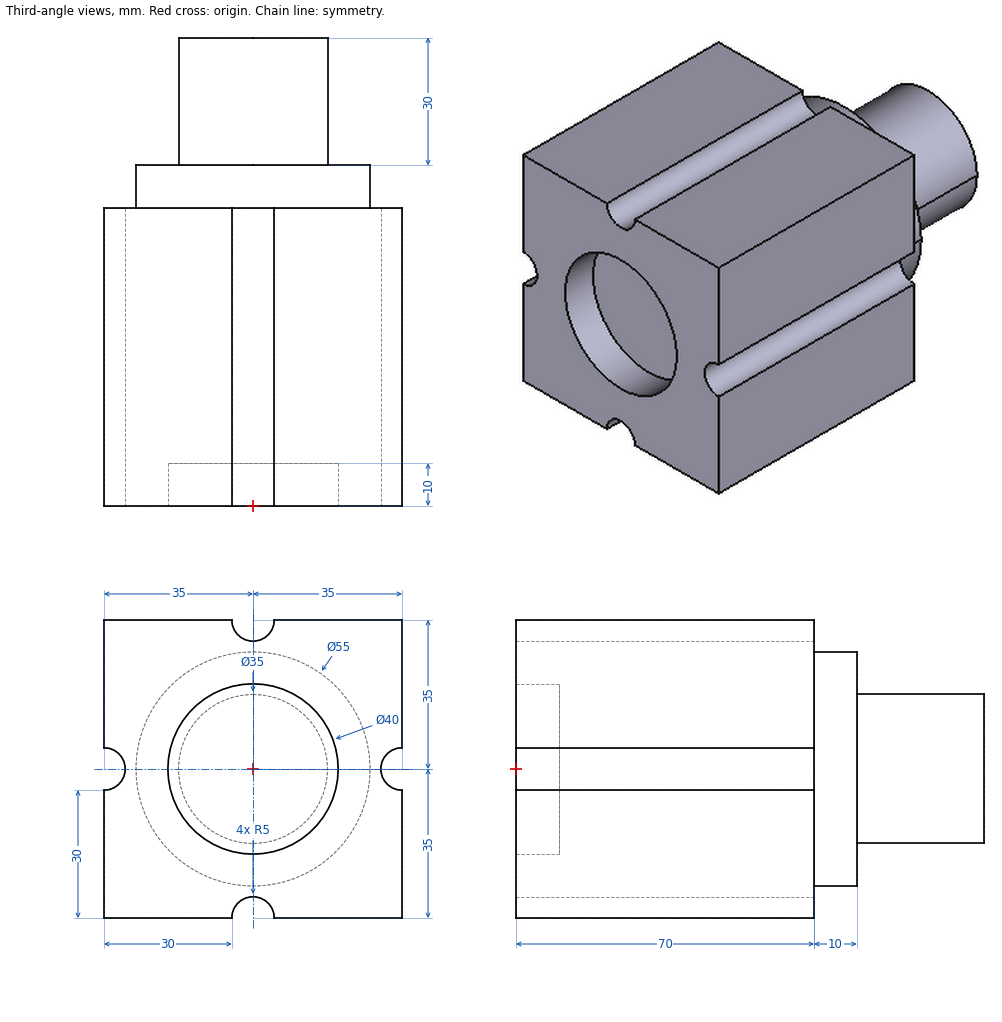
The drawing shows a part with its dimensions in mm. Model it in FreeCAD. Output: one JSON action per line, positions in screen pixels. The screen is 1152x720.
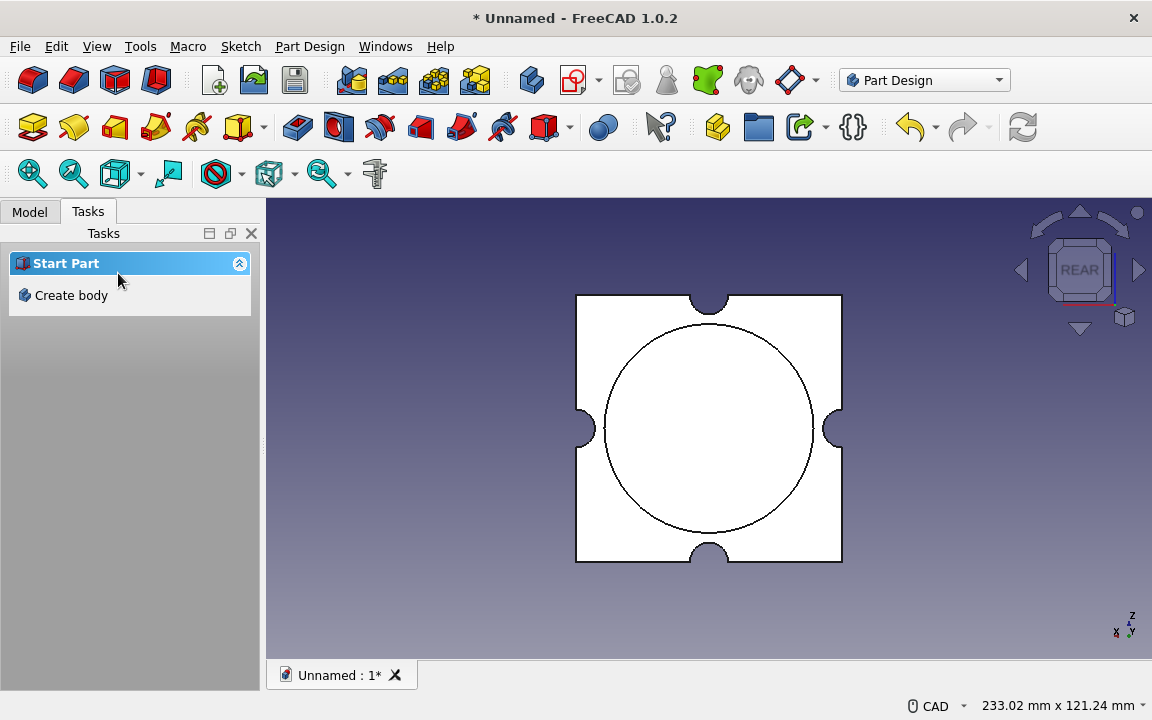
{"action": "left_click", "coordinate": [709, 428]}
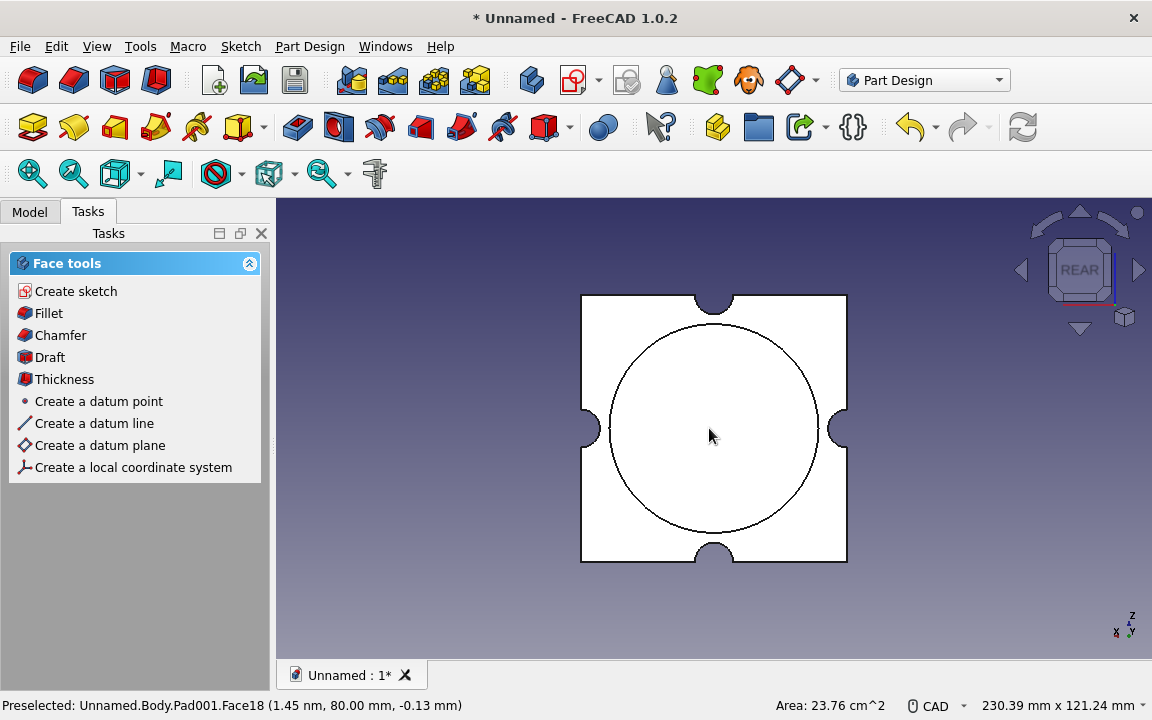
{"action": "left_click", "coordinate": [572, 80]}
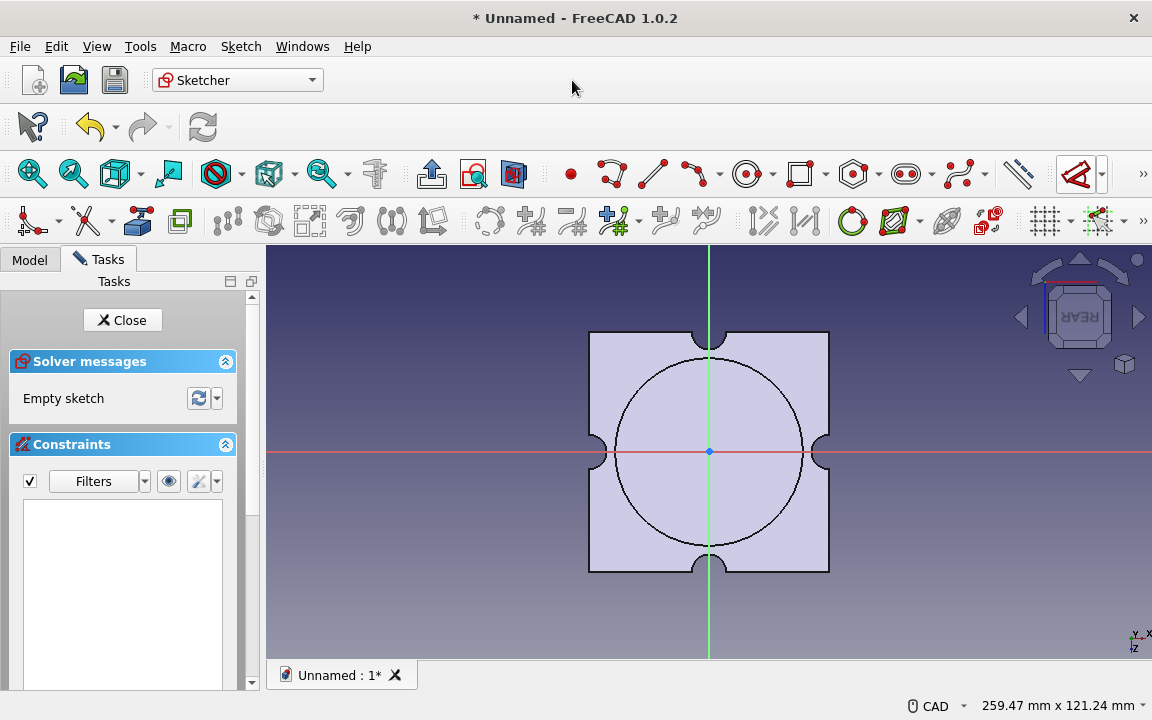
{"action": "scroll", "coordinate": [765, 452], "scroll_direction": "up", "scroll_amount": 4}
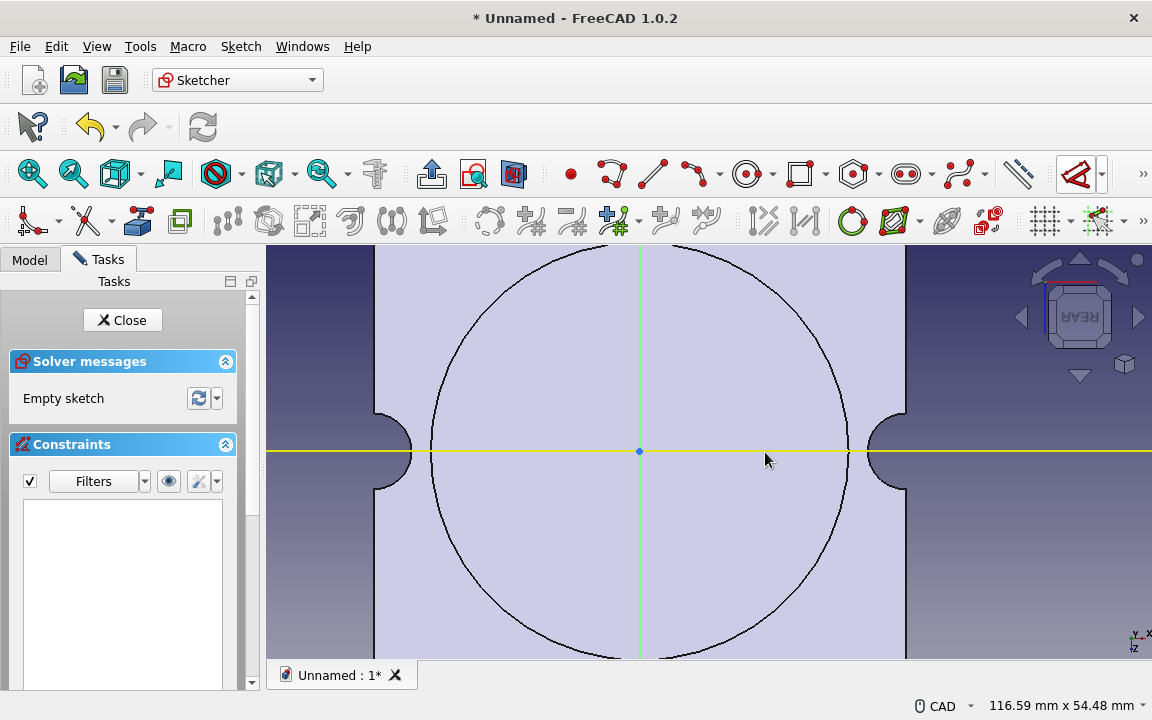
{"action": "left_click", "coordinate": [746, 174]}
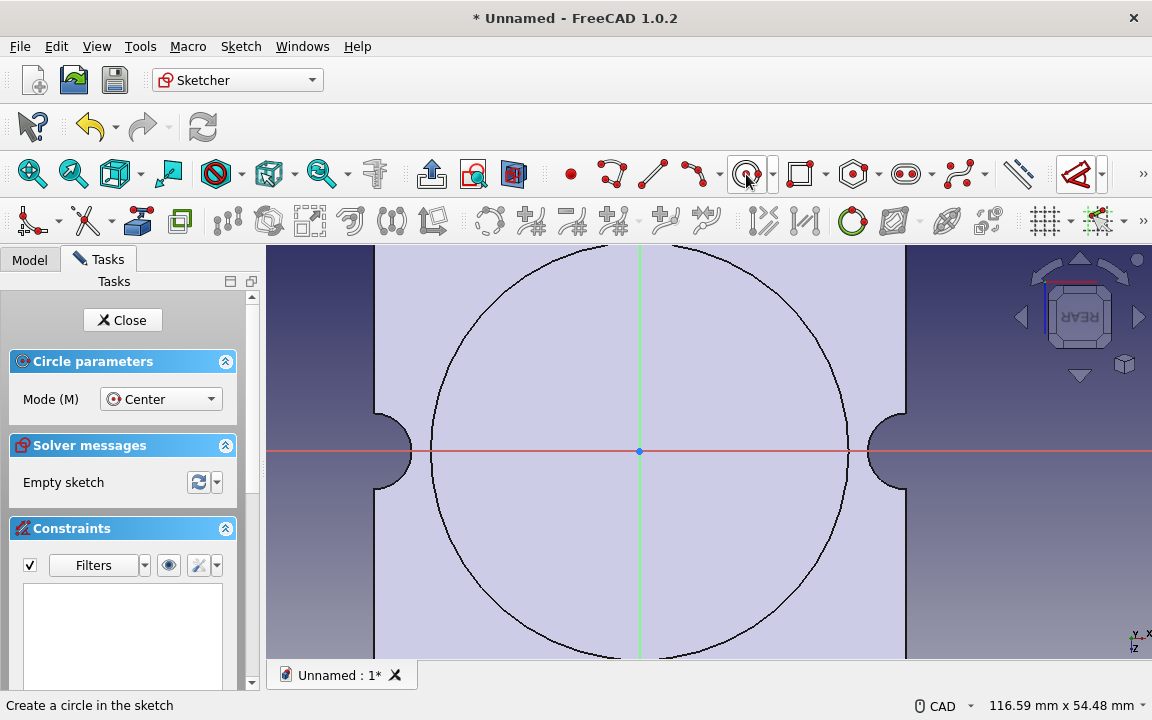
{"action": "left_click", "coordinate": [640, 451]}
{"action": "mouse_move", "coordinate": [734, 357]}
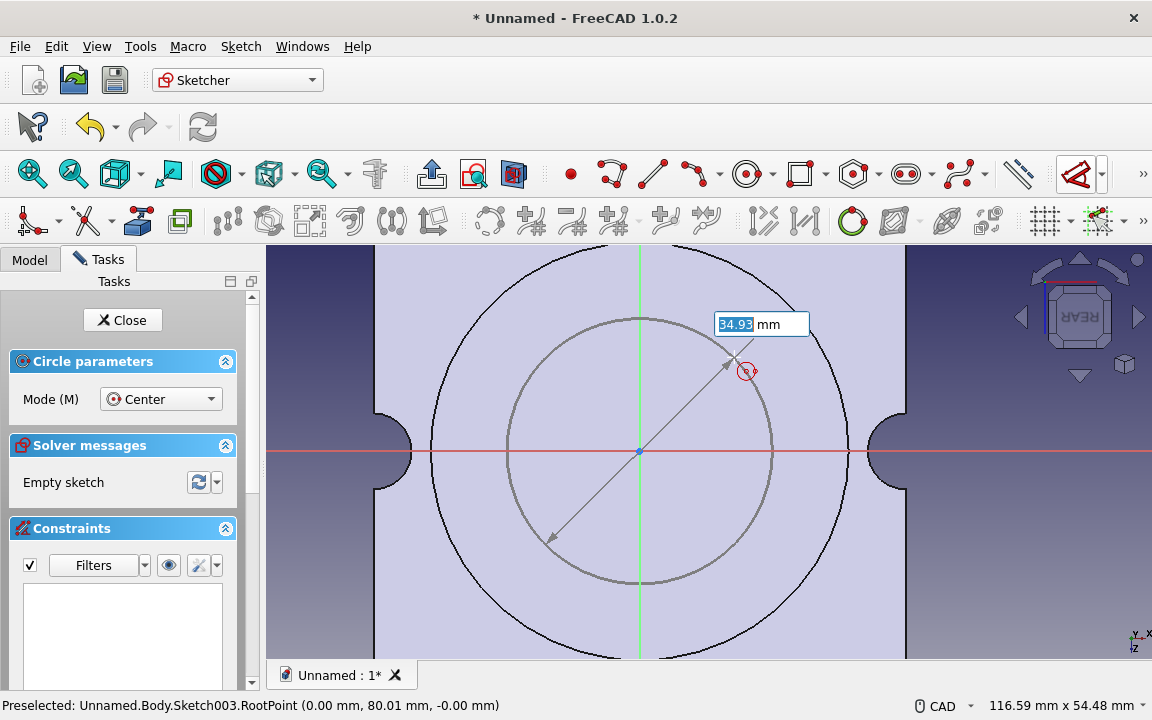
{"action": "type", "text": "35"}
{"action": "key", "text": "Return"}
{"action": "key", "text": "Escape"}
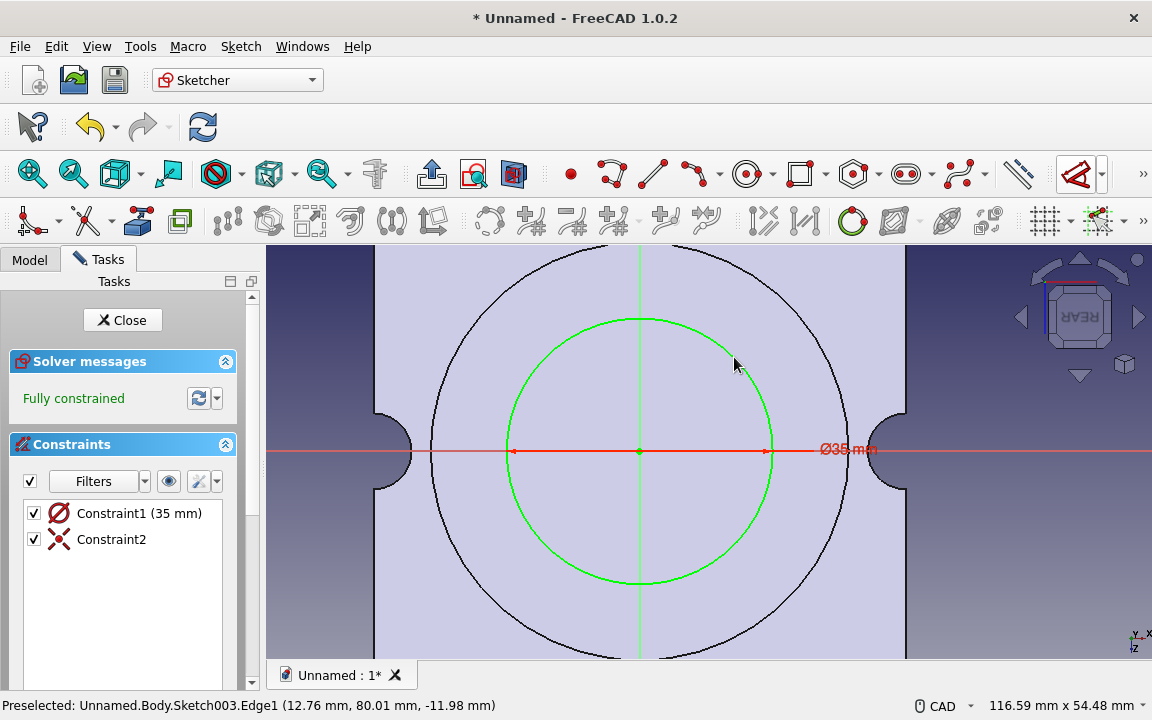
{"action": "left_click", "coordinate": [123, 320]}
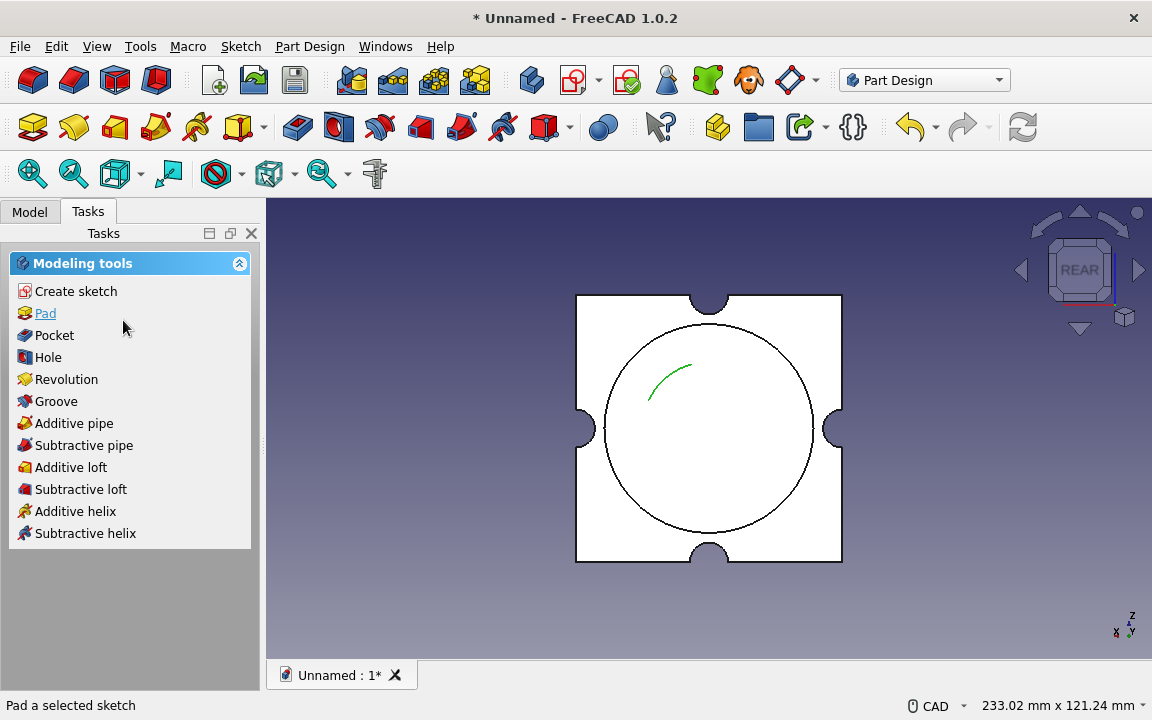
{"action": "left_click", "coordinate": [33, 128]}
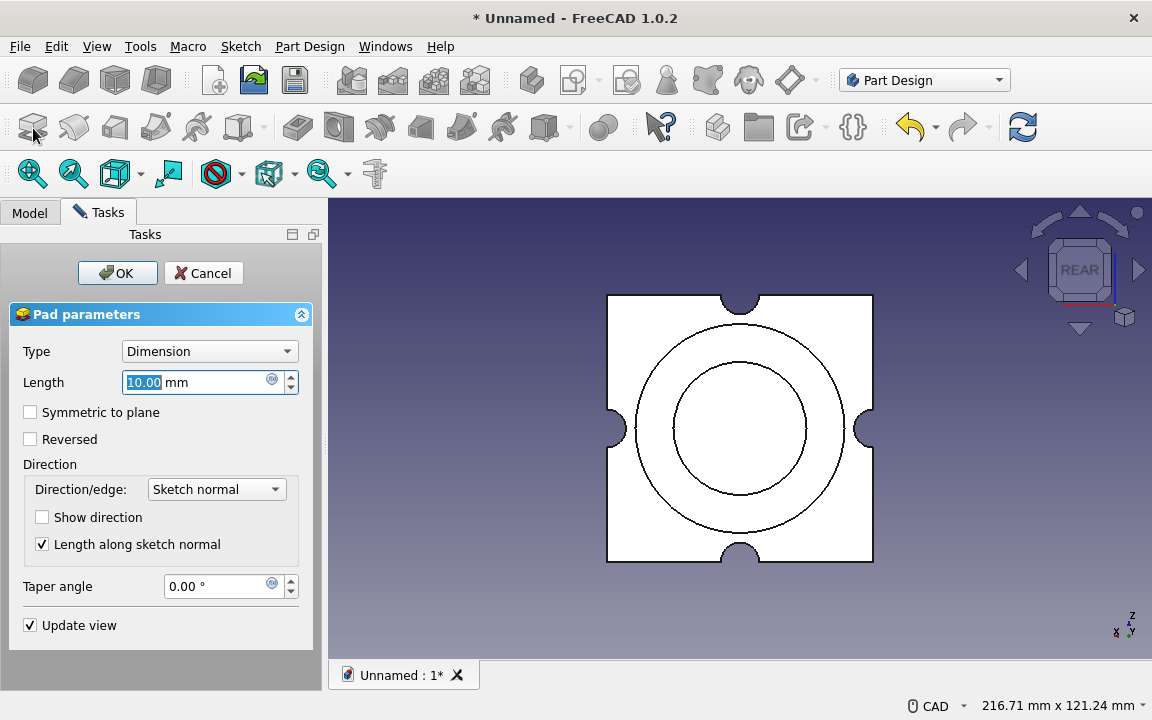
{"action": "type", "text": "30"}
{"action": "key", "text": "Tab"}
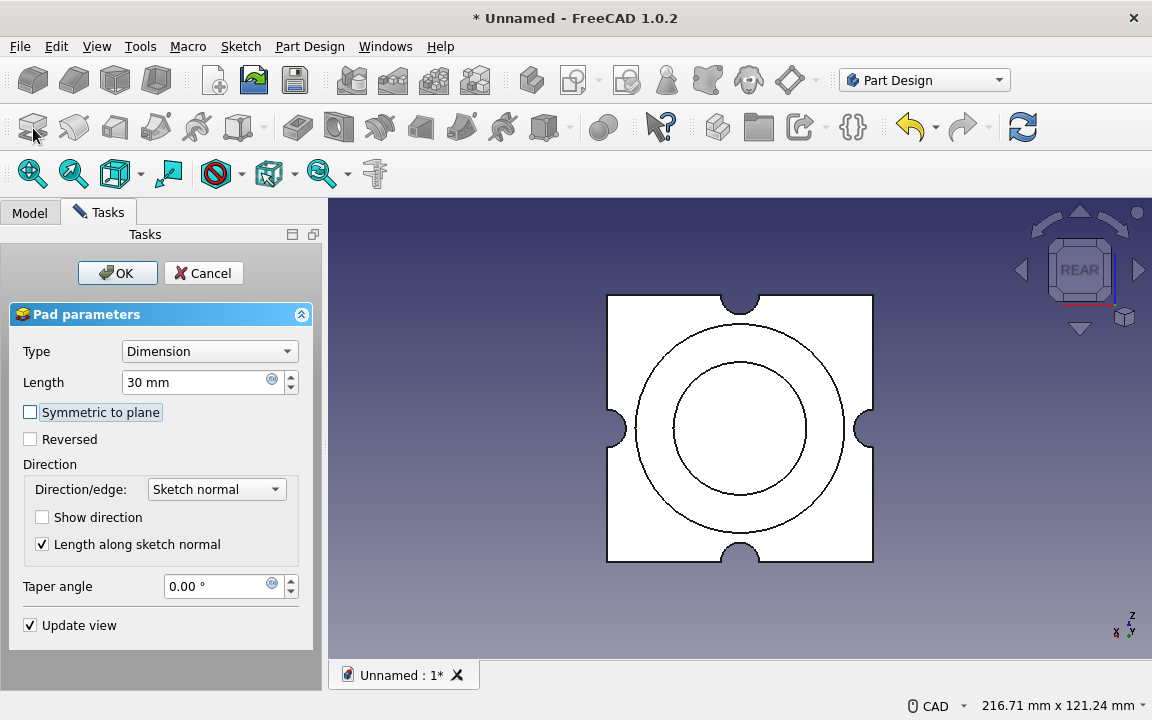
{"action": "left_click", "coordinate": [118, 273]}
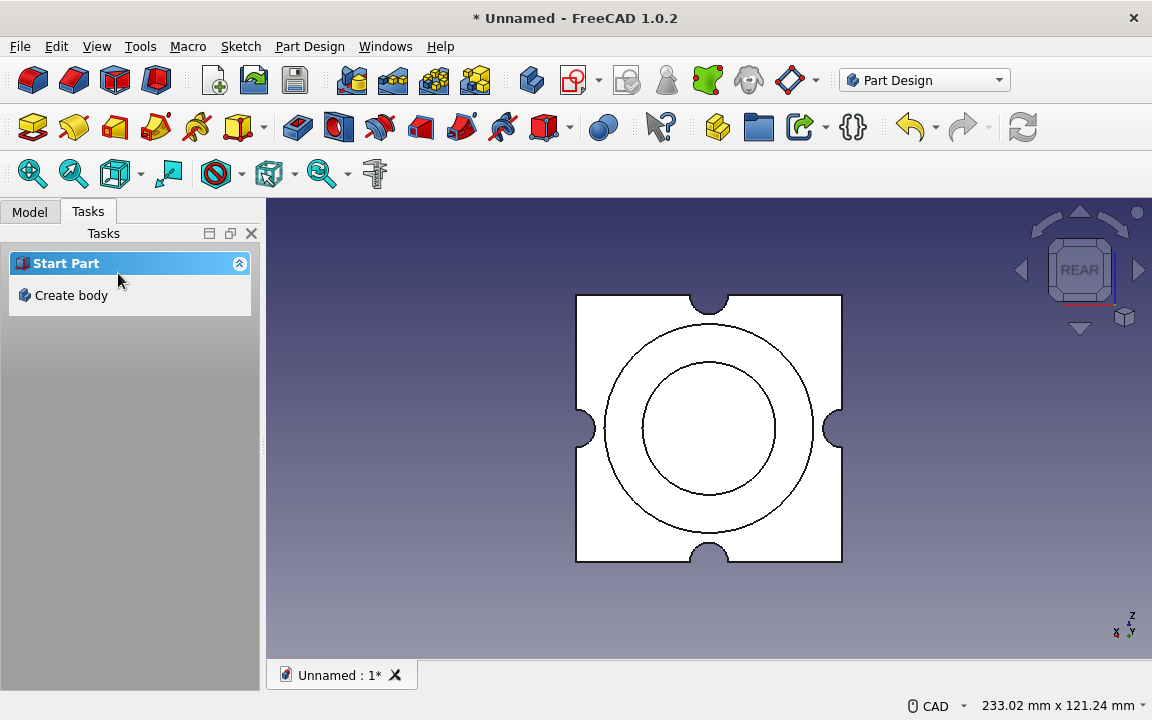
{"action": "key", "text": "0"}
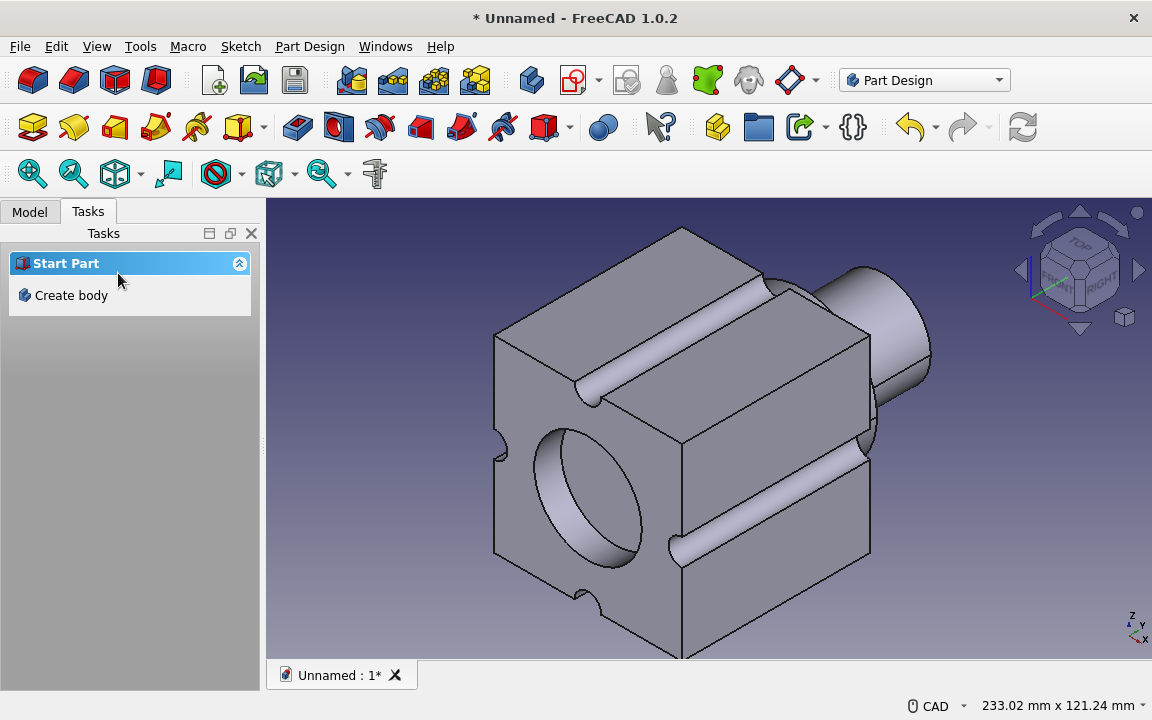
{"action": "left_click", "coordinate": [33, 174]}